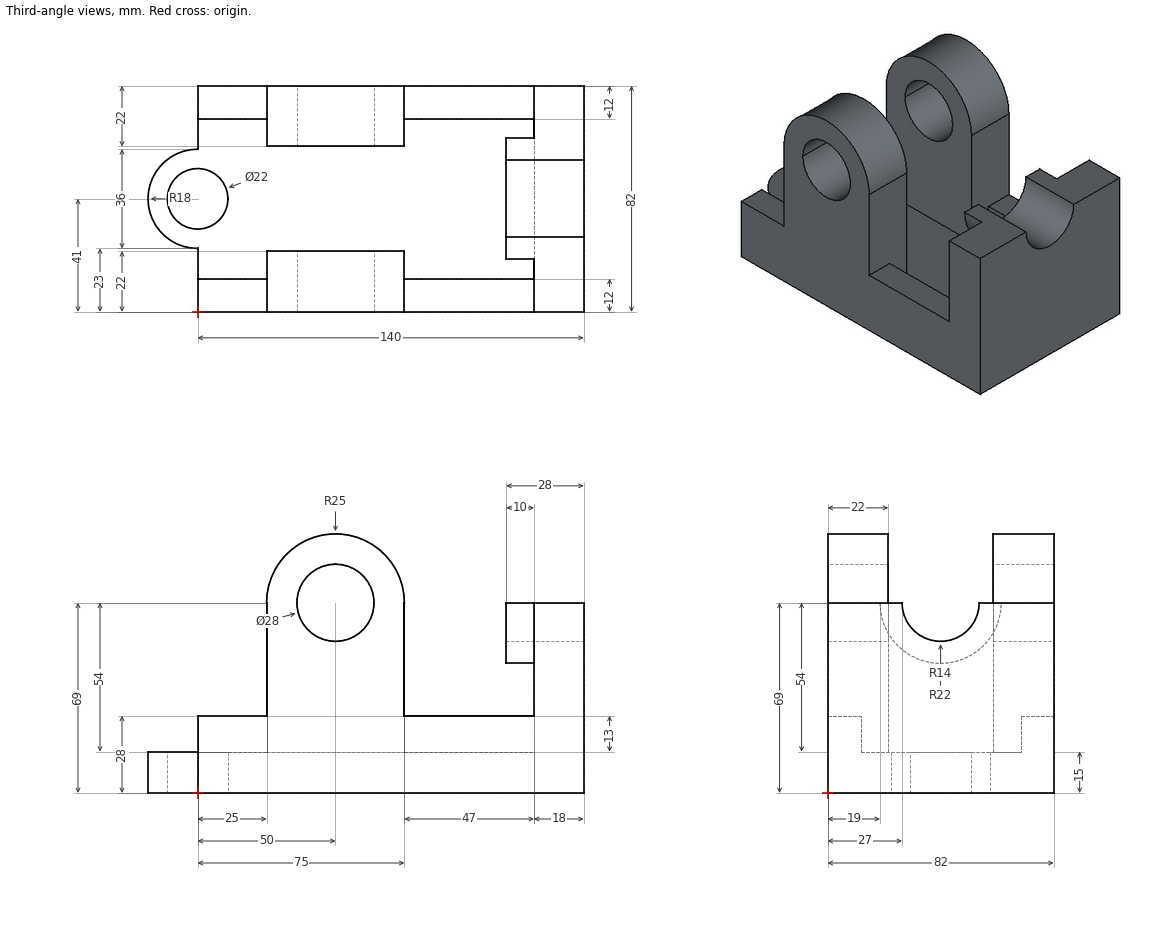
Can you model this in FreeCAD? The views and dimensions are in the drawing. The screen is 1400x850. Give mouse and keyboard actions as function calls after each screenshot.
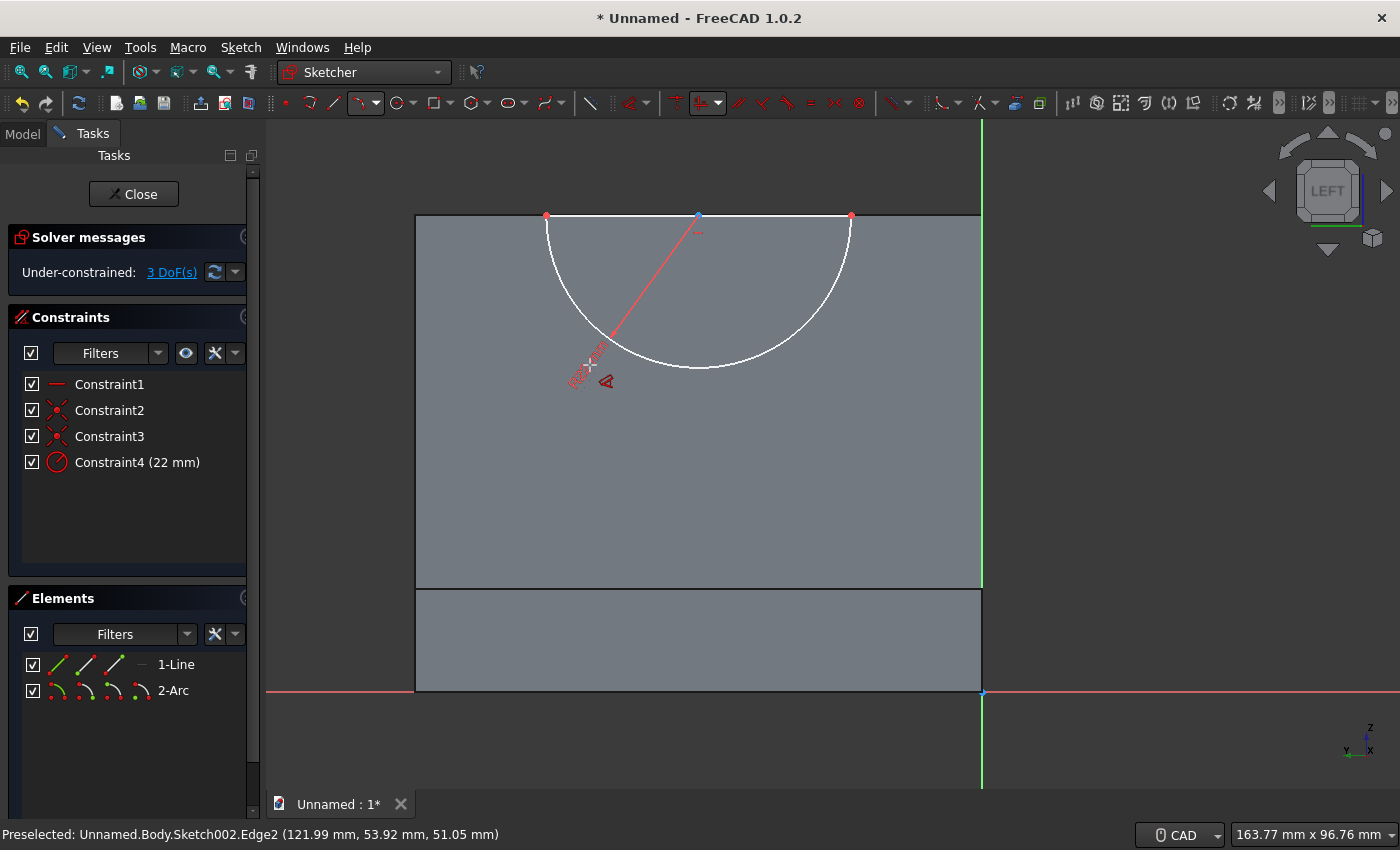
click(851, 216)
click(917, 726)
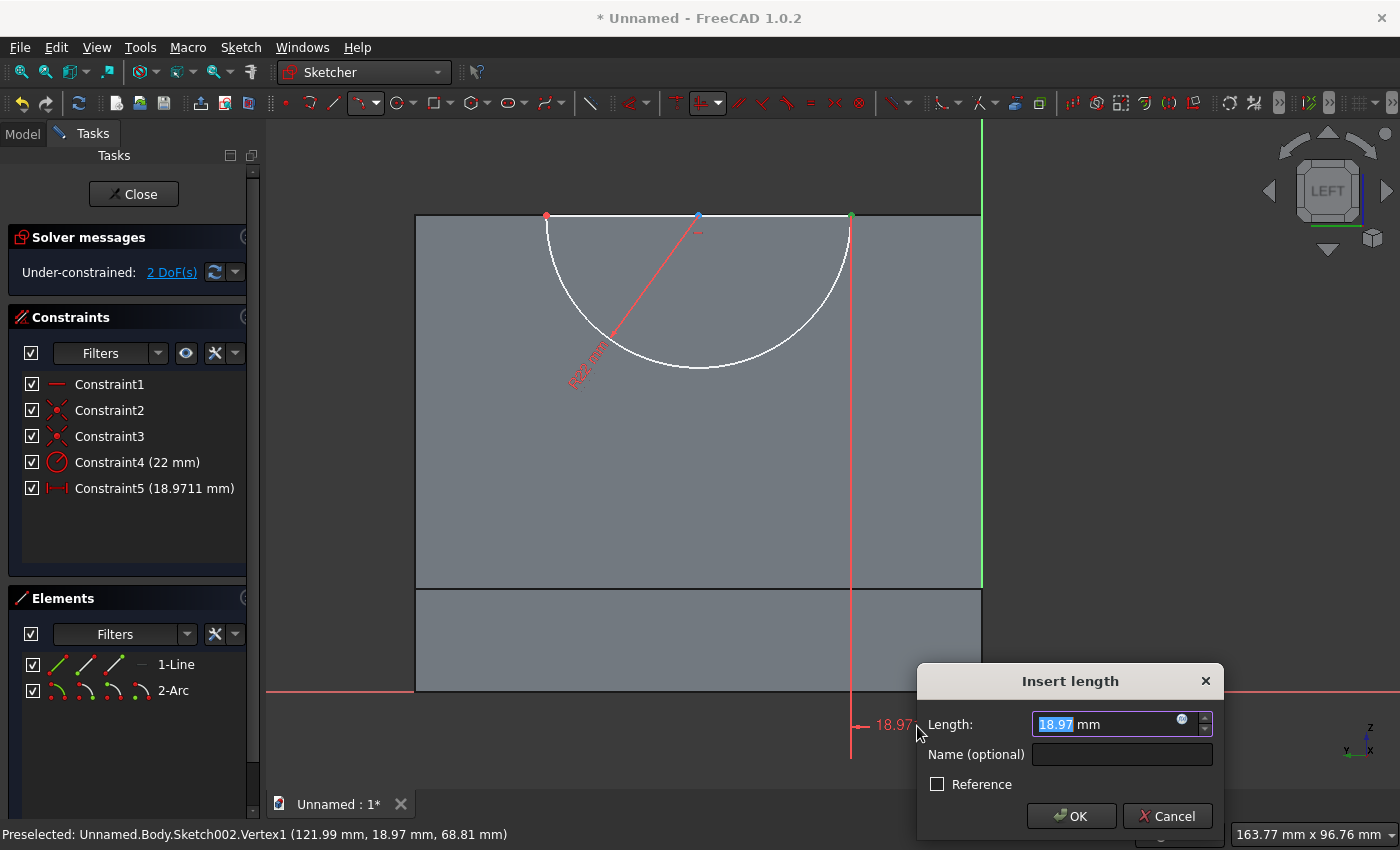
text(19)
key(Return)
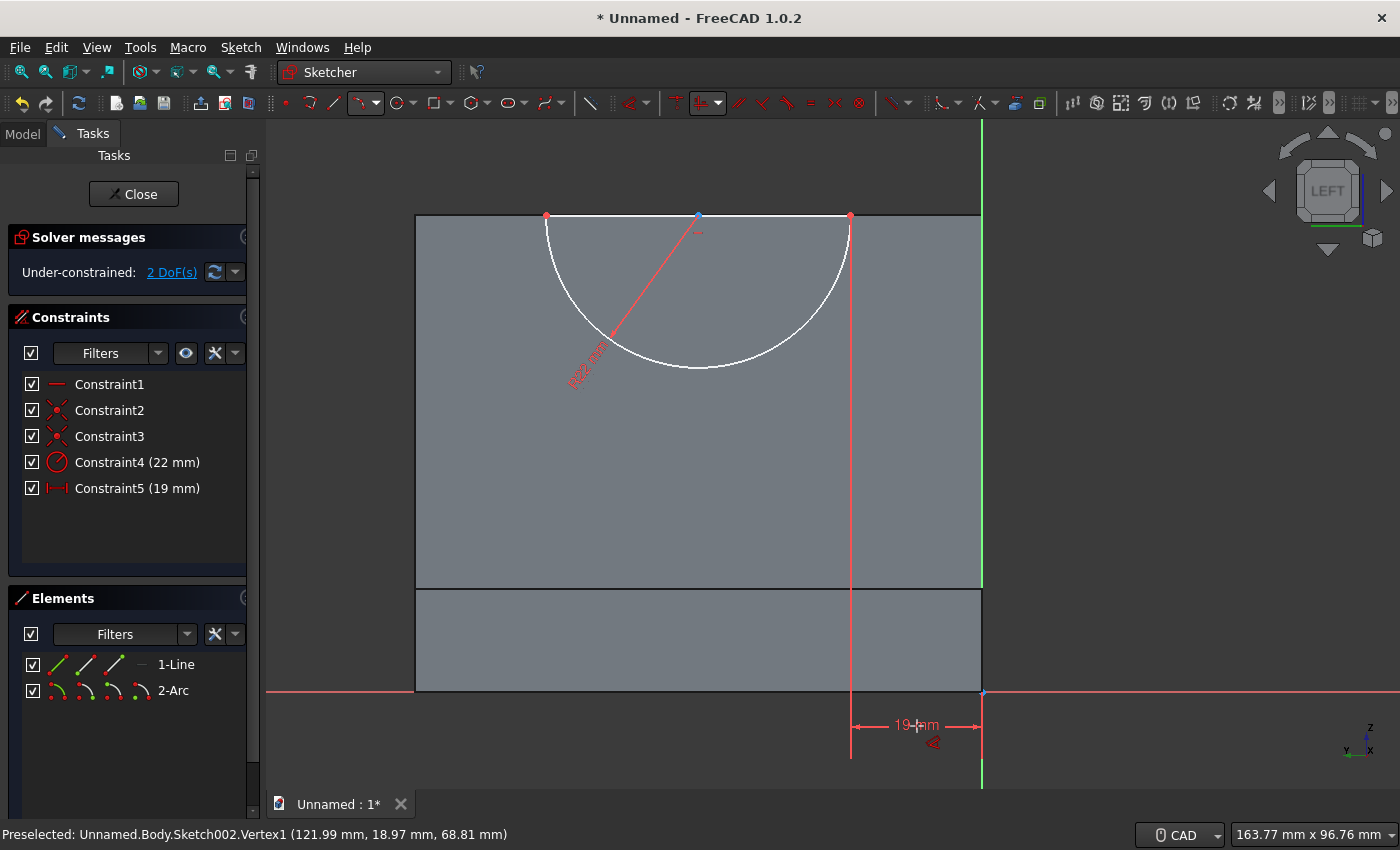
click(851, 216)
click(1016, 454)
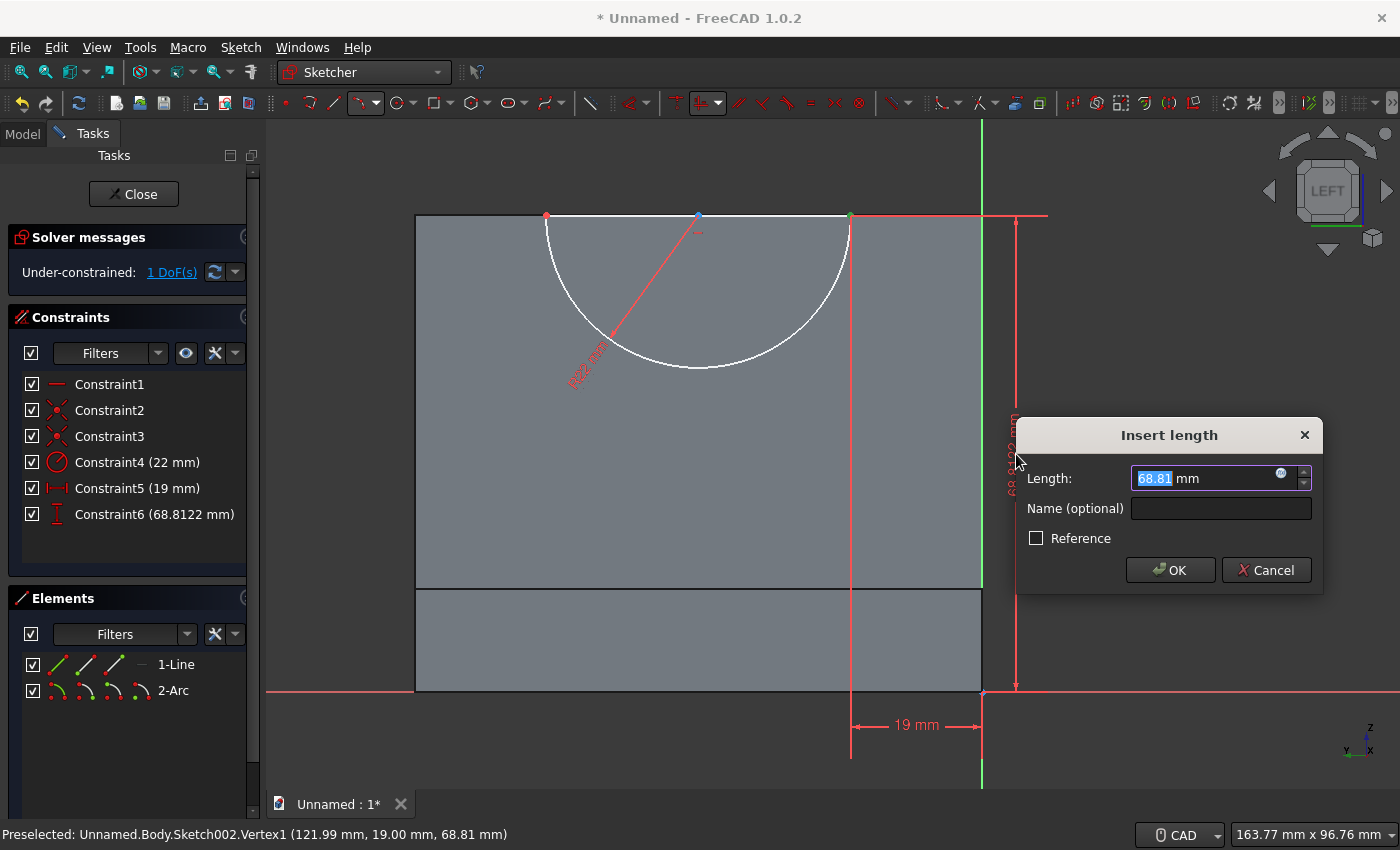
text(69)
key(Return)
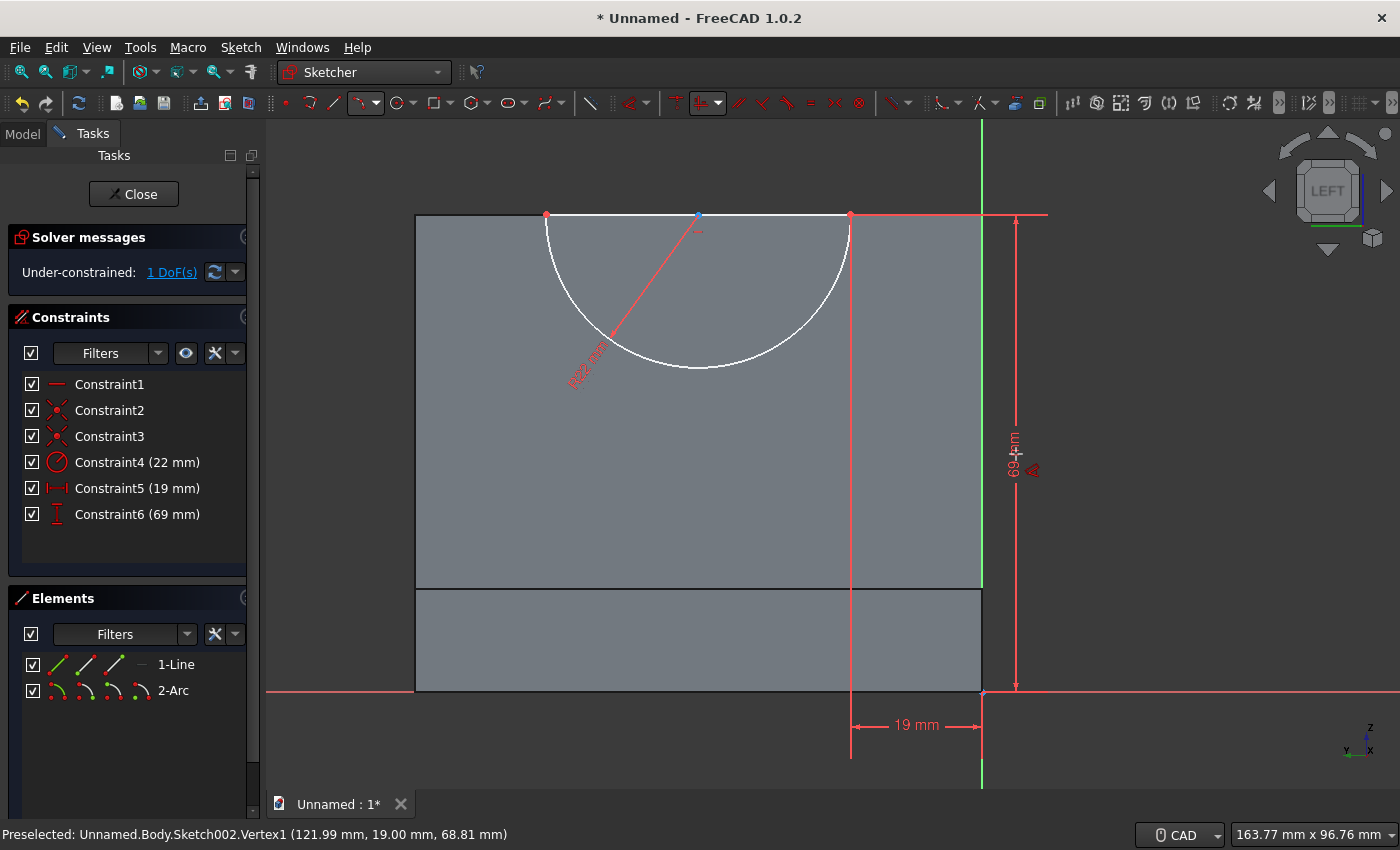
click(698, 216)
click(1016, 344)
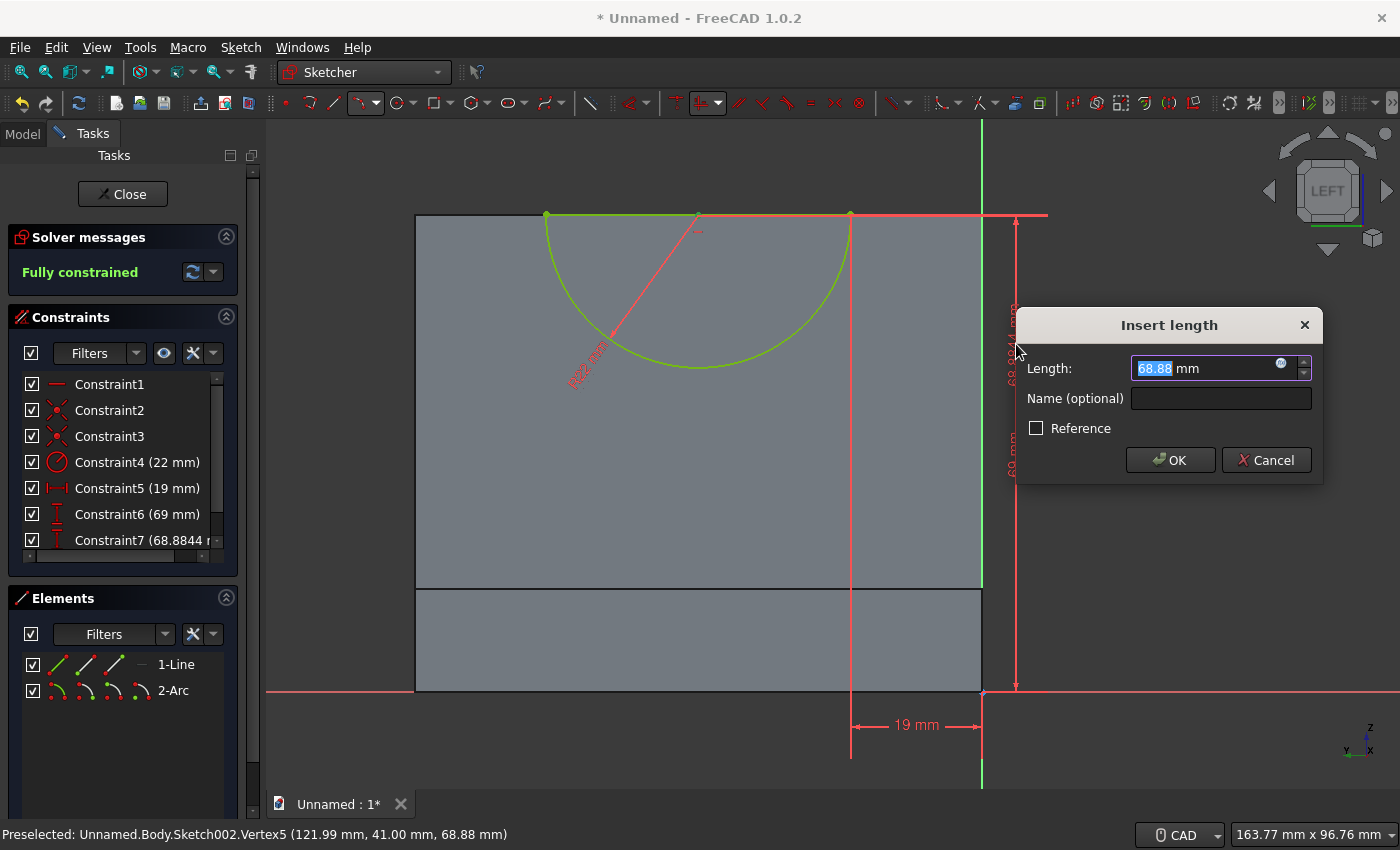
text(69)
key(Return)
key(Escape)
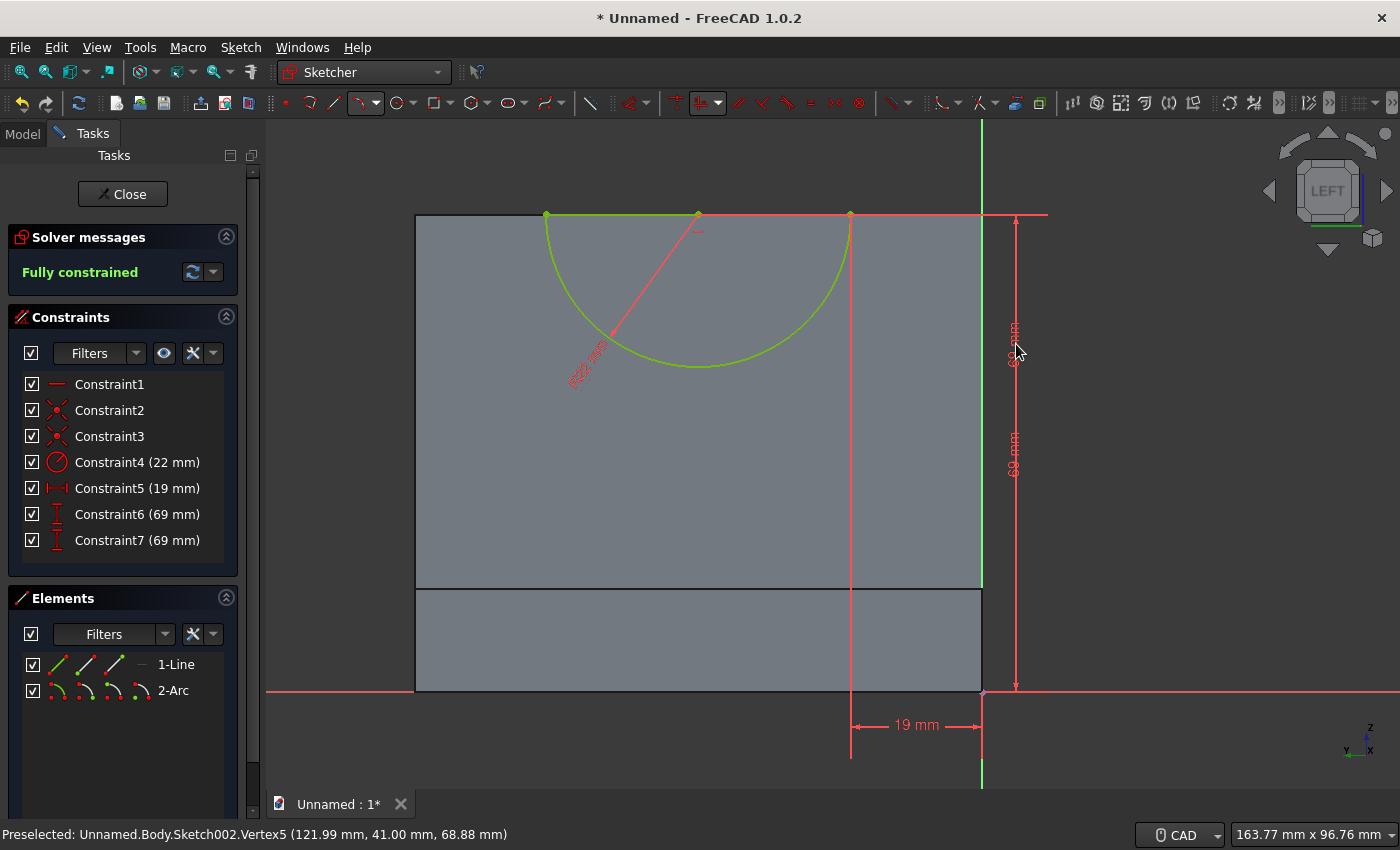
click(123, 194)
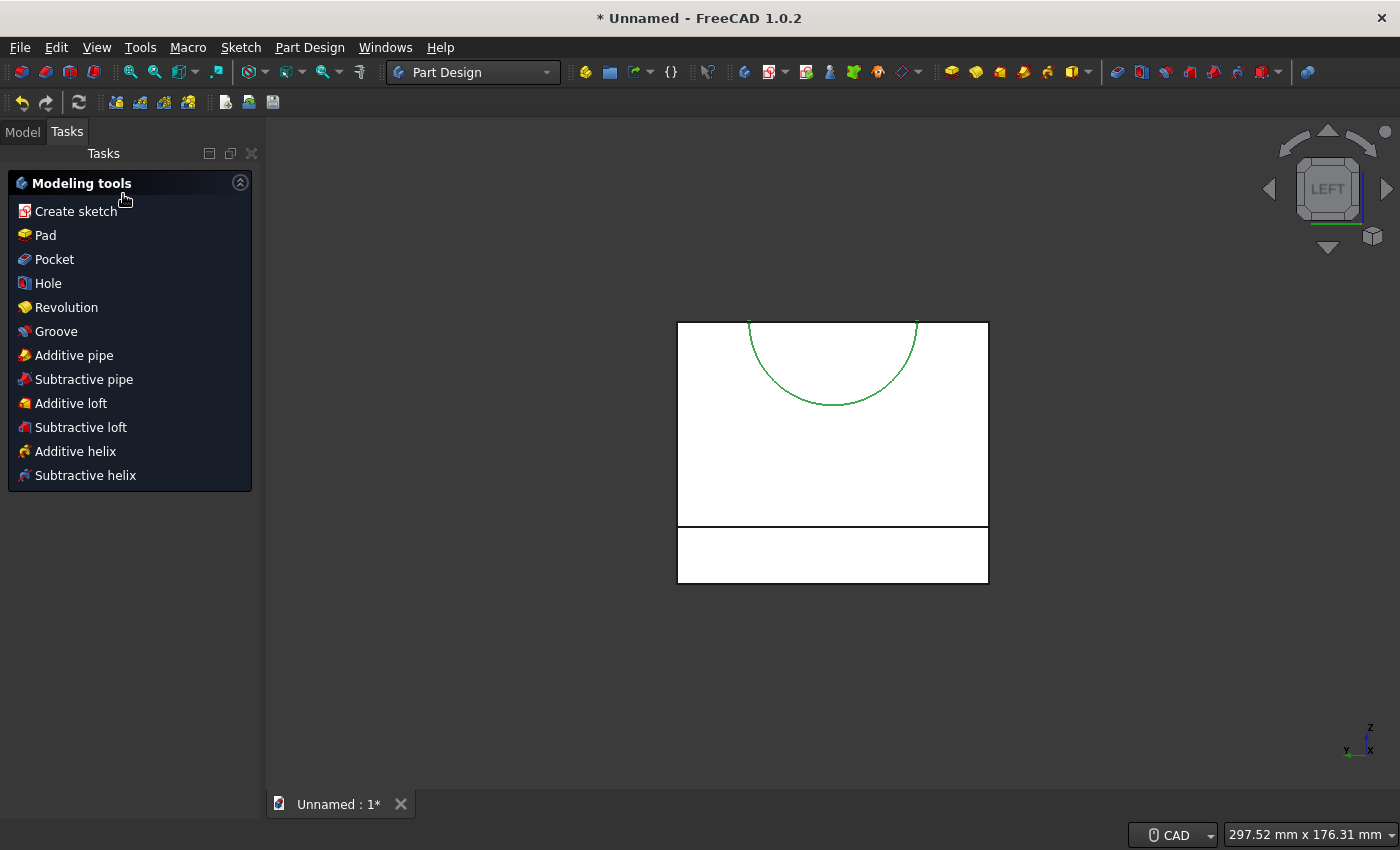
click(952, 72)